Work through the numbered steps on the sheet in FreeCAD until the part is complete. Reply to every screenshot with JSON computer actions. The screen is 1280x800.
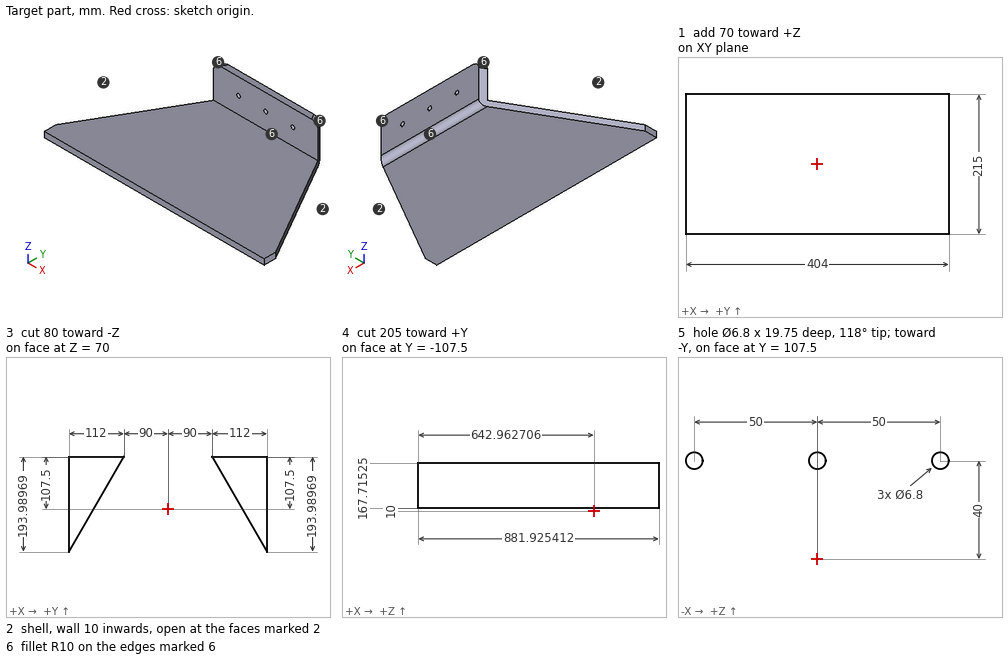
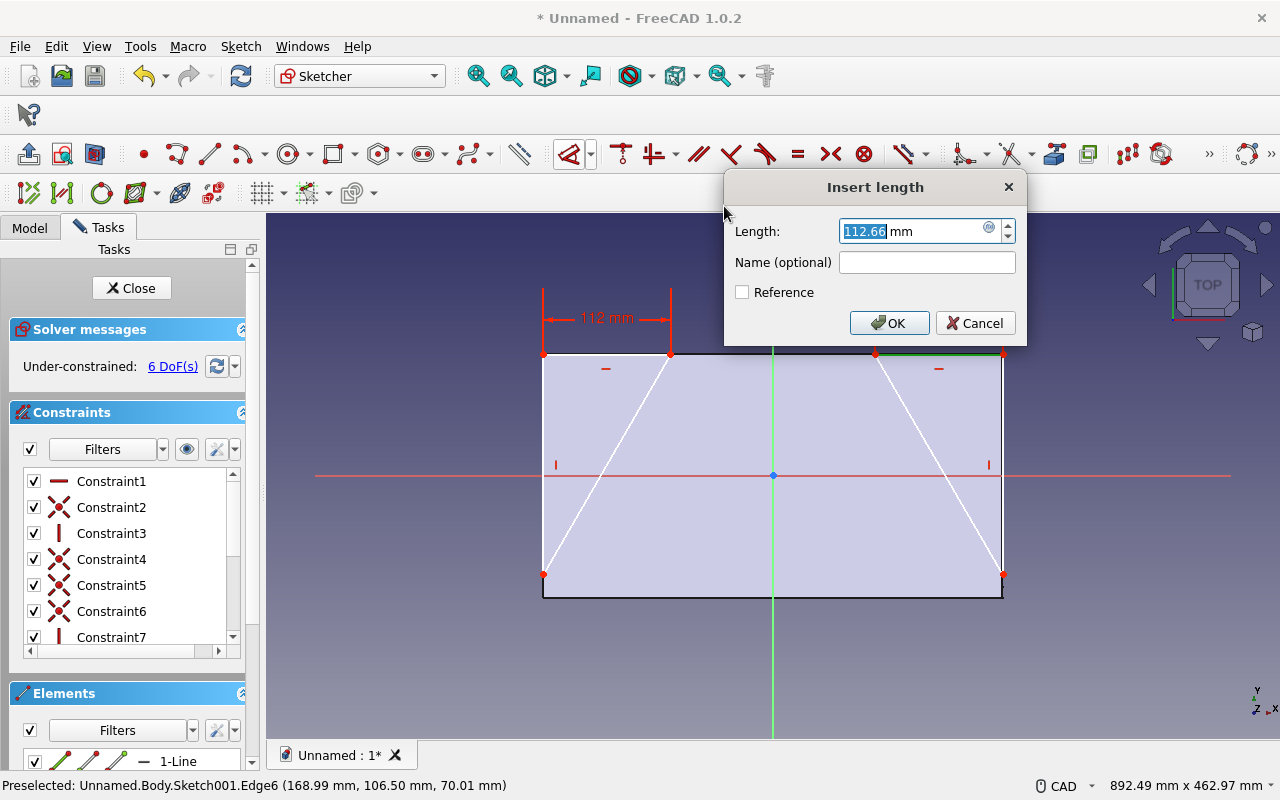
{"action": "type", "text": "112"}
{"action": "key", "text": "Return"}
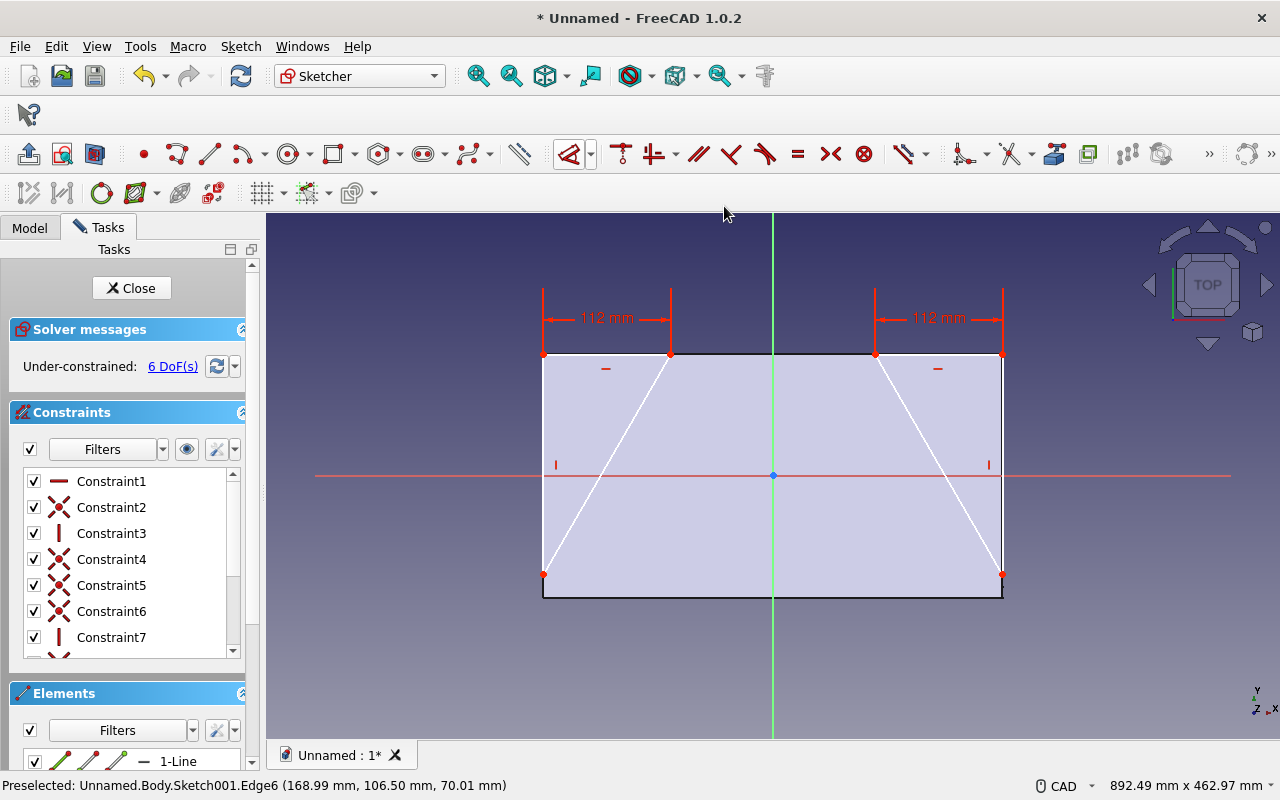
{"action": "left_click", "coordinate": [671, 355]}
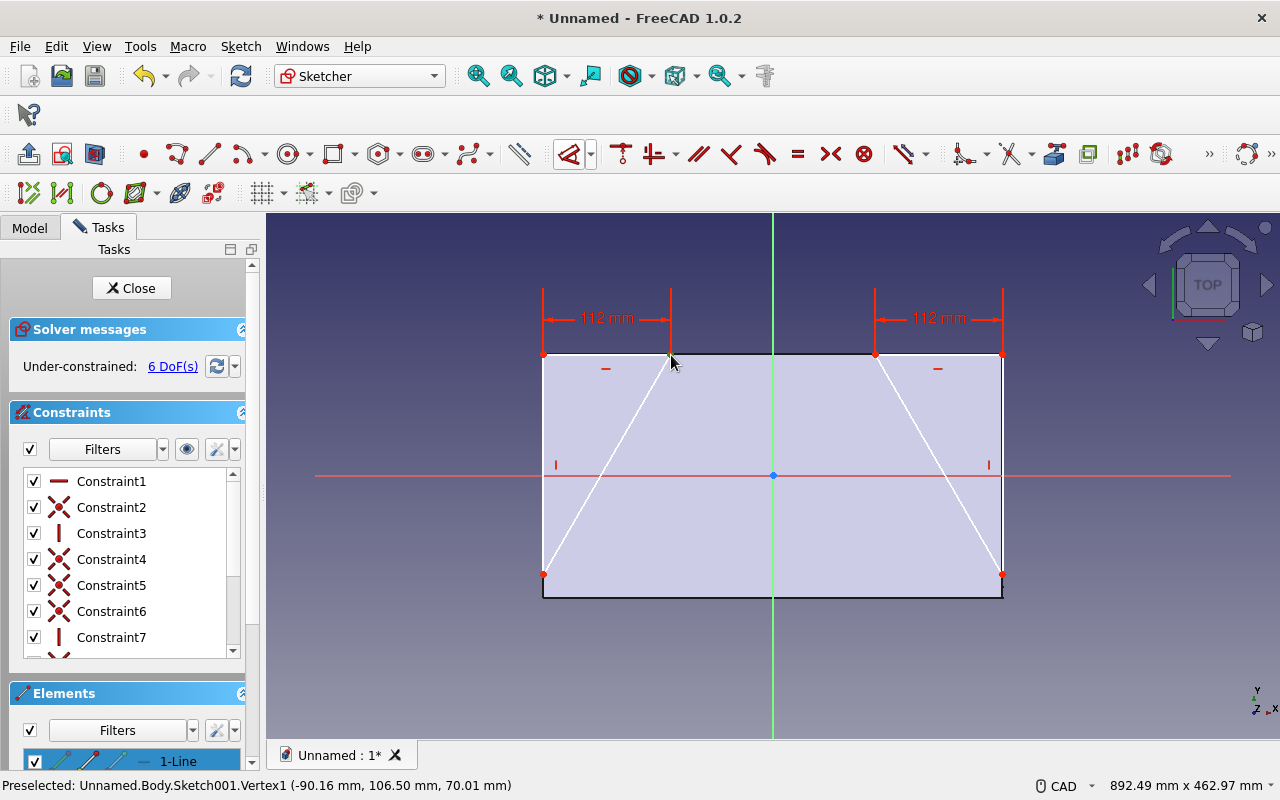
{"action": "left_click", "coordinate": [590, 154]}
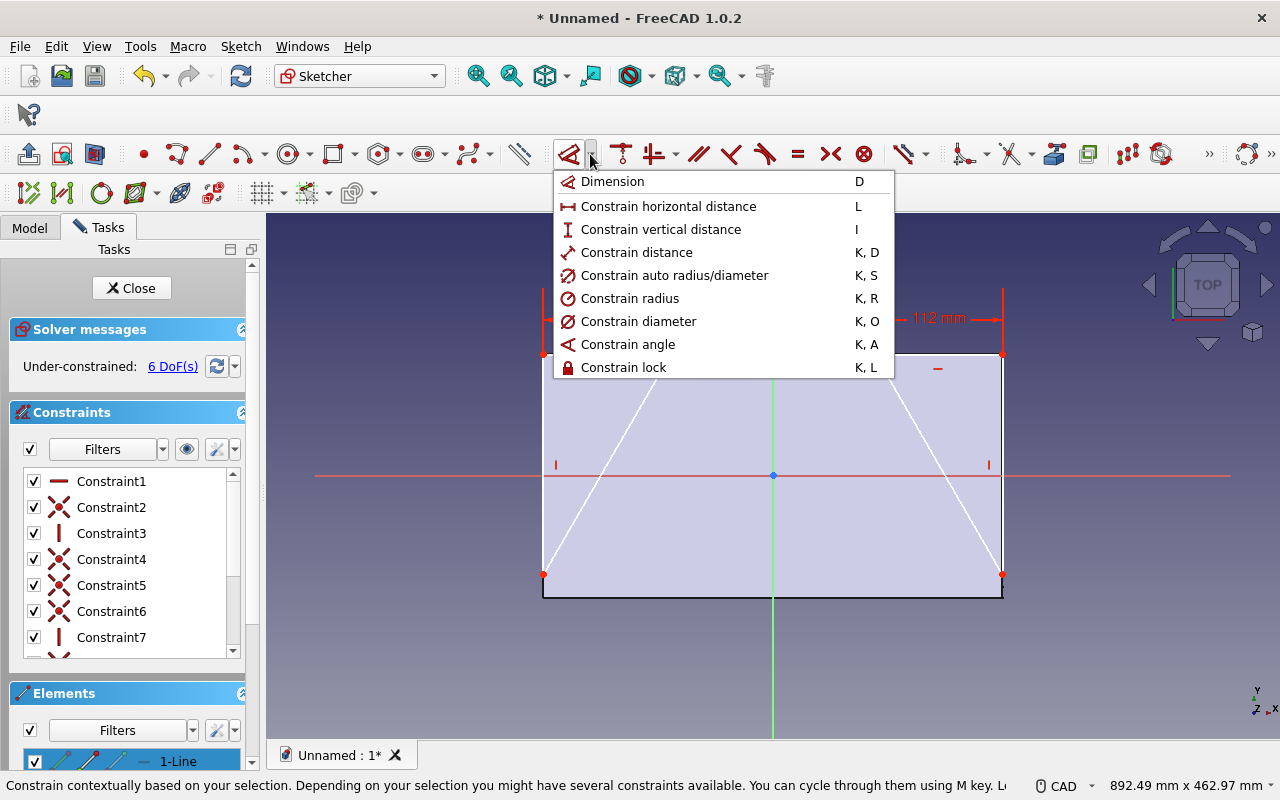
{"action": "left_click", "coordinate": [724, 206]}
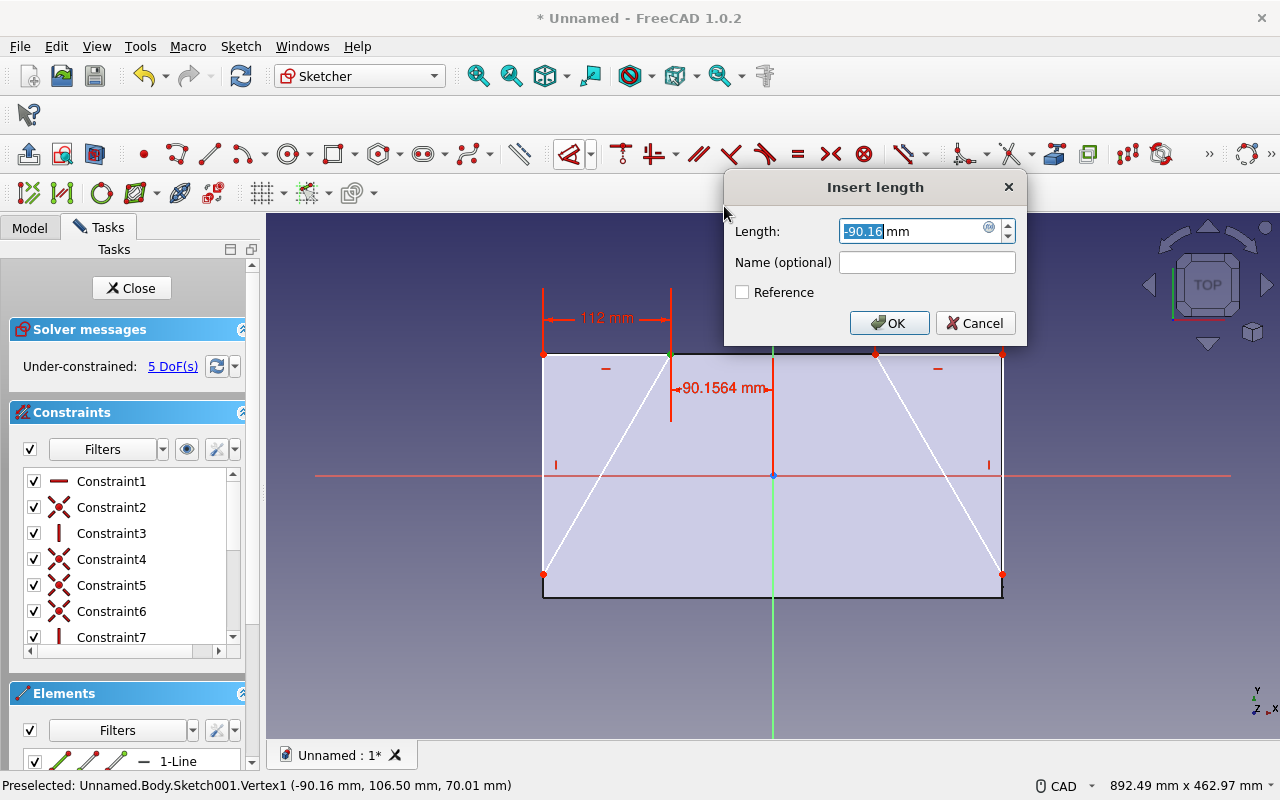
{"action": "type", "text": "-90"}
{"action": "key", "text": "Return"}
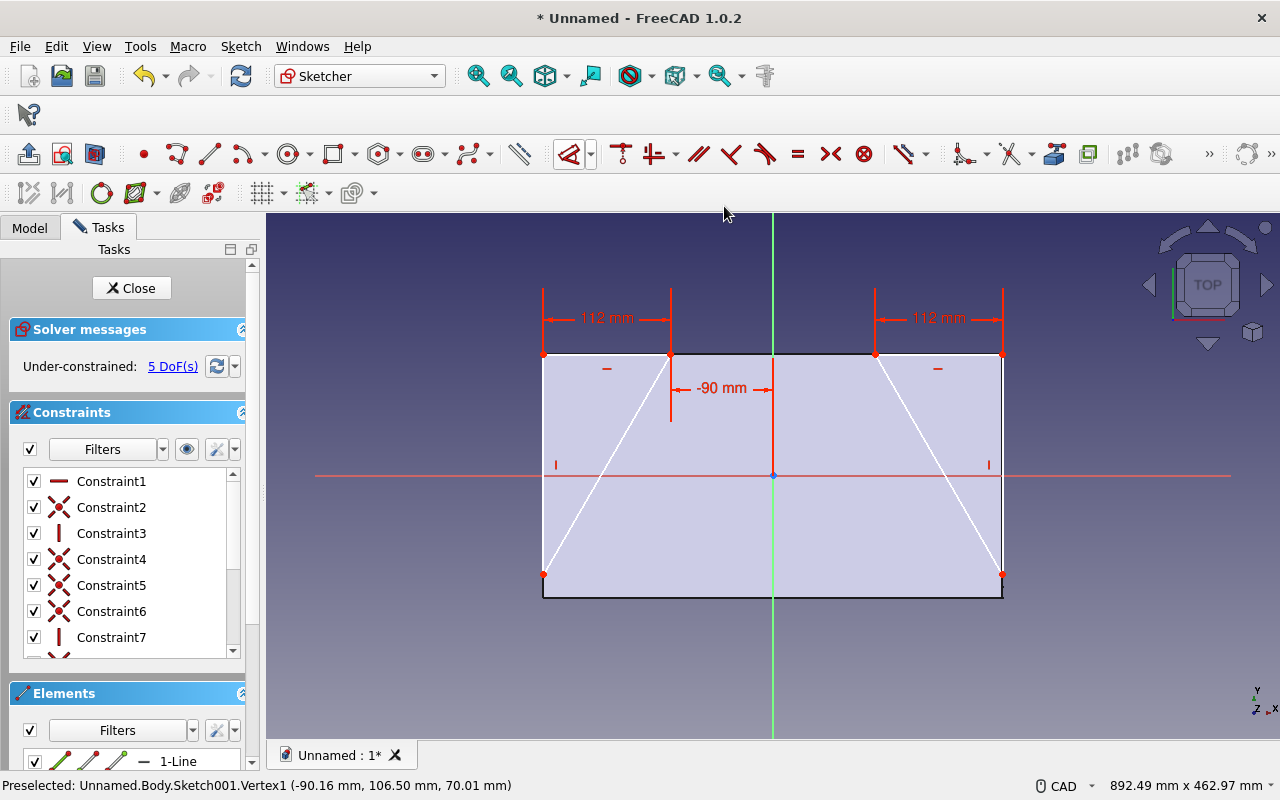
{"action": "left_click", "coordinate": [875, 355]}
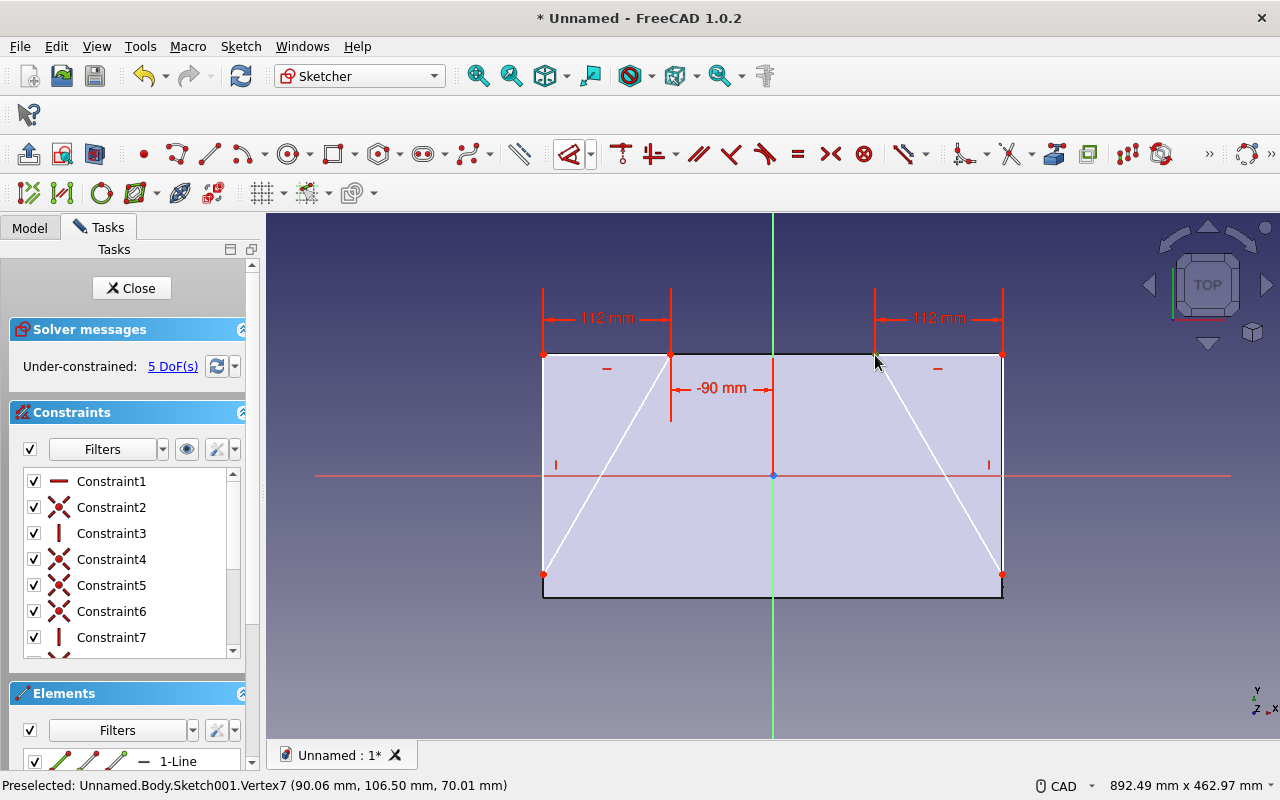
{"action": "left_click", "coordinate": [590, 154]}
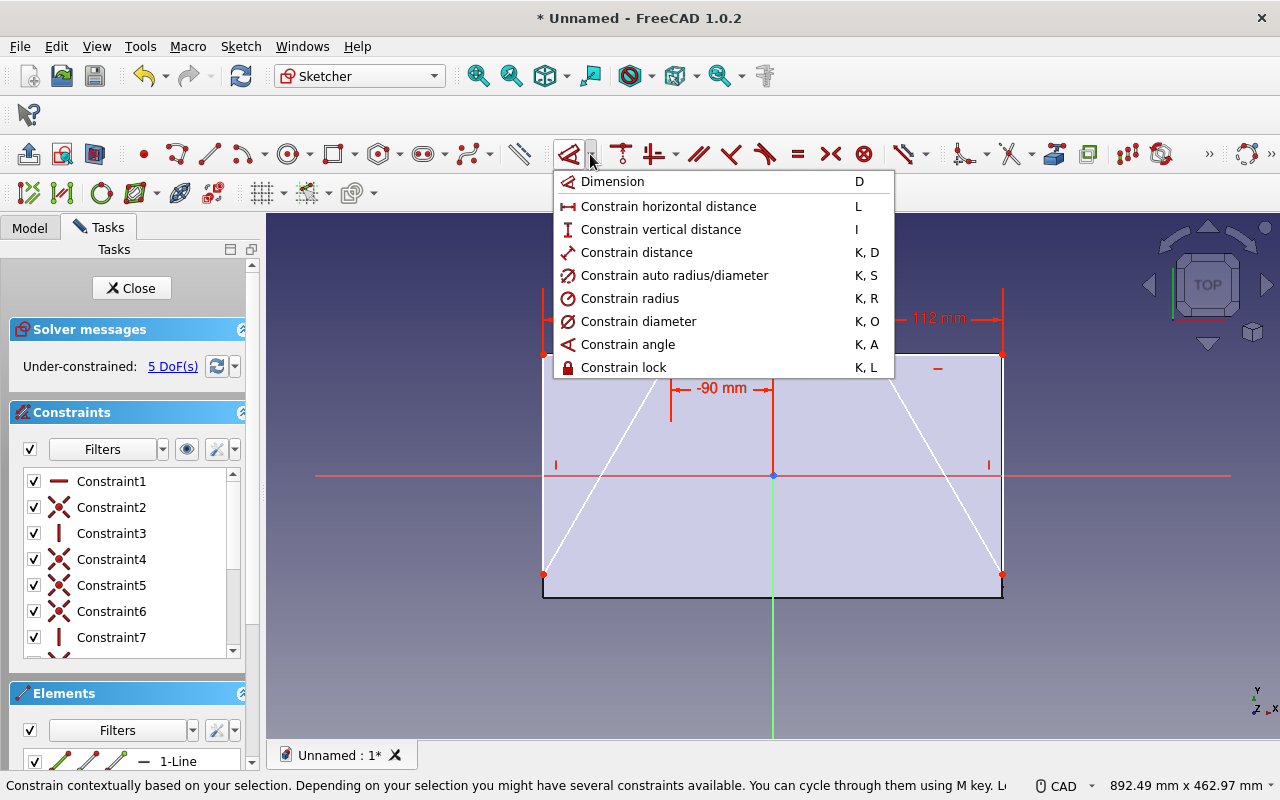
{"action": "left_click", "coordinate": [724, 206]}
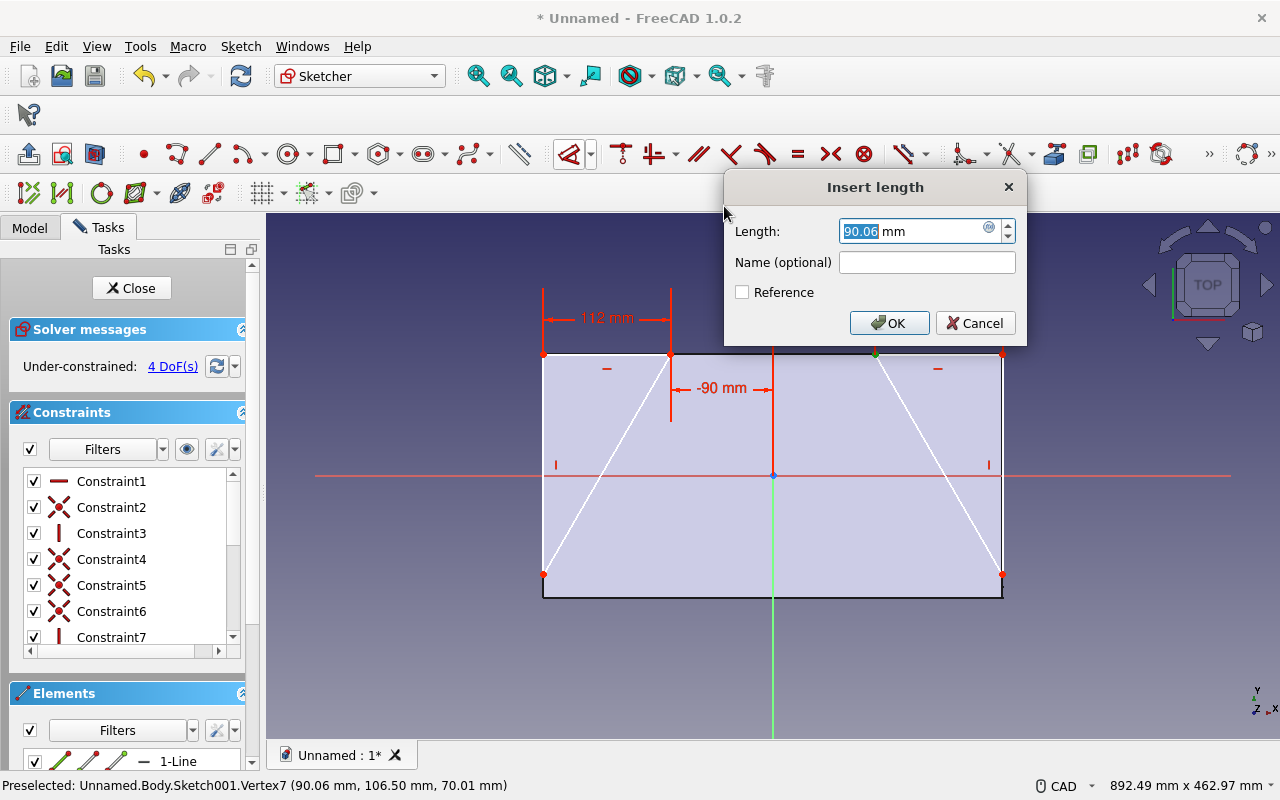
{"action": "type", "text": "90"}
{"action": "key", "text": "Return"}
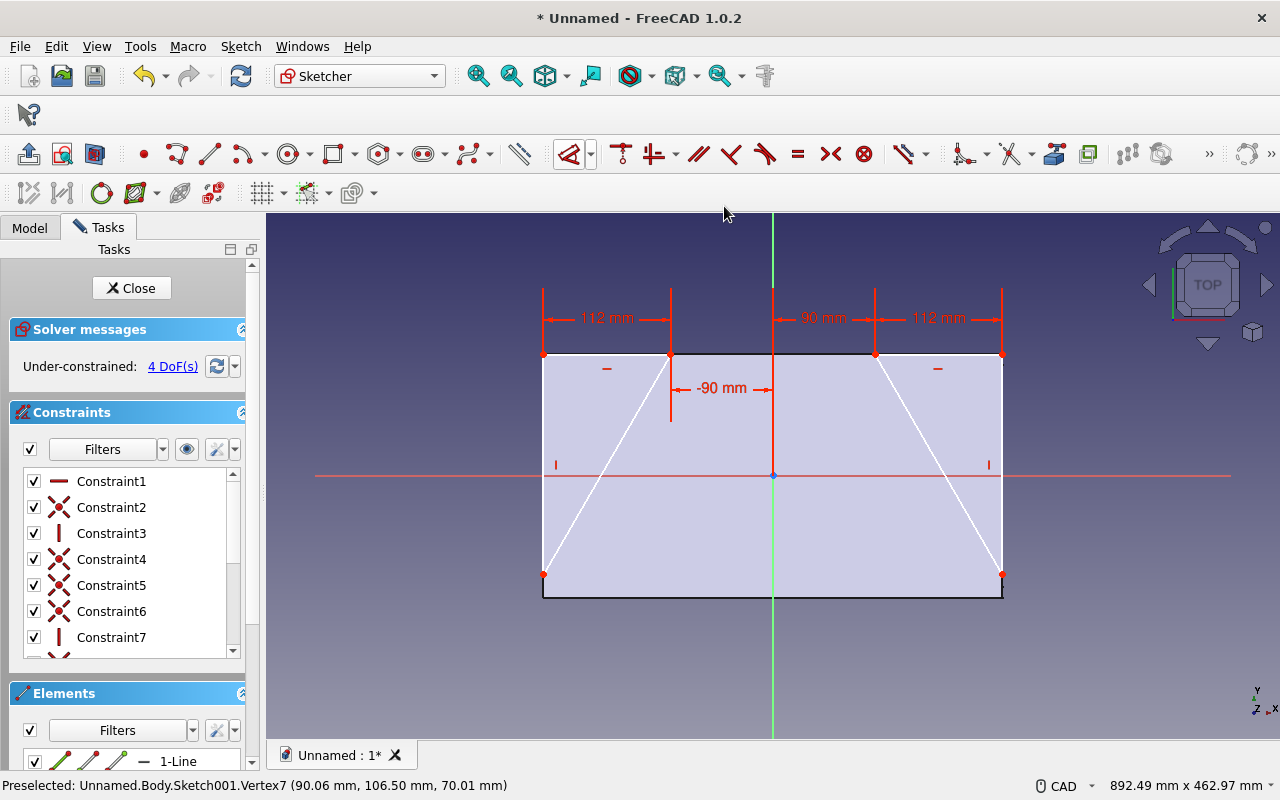
{"action": "left_click", "coordinate": [671, 355]}